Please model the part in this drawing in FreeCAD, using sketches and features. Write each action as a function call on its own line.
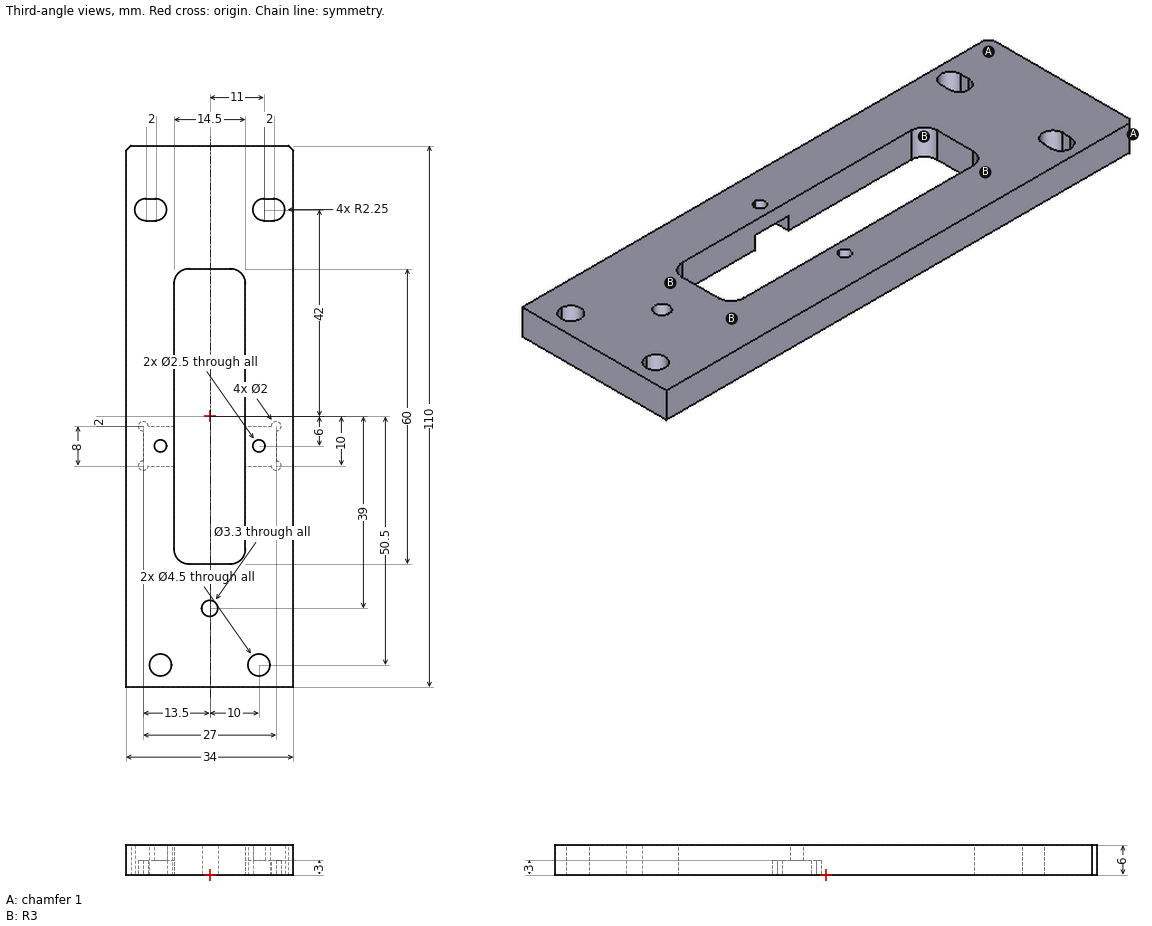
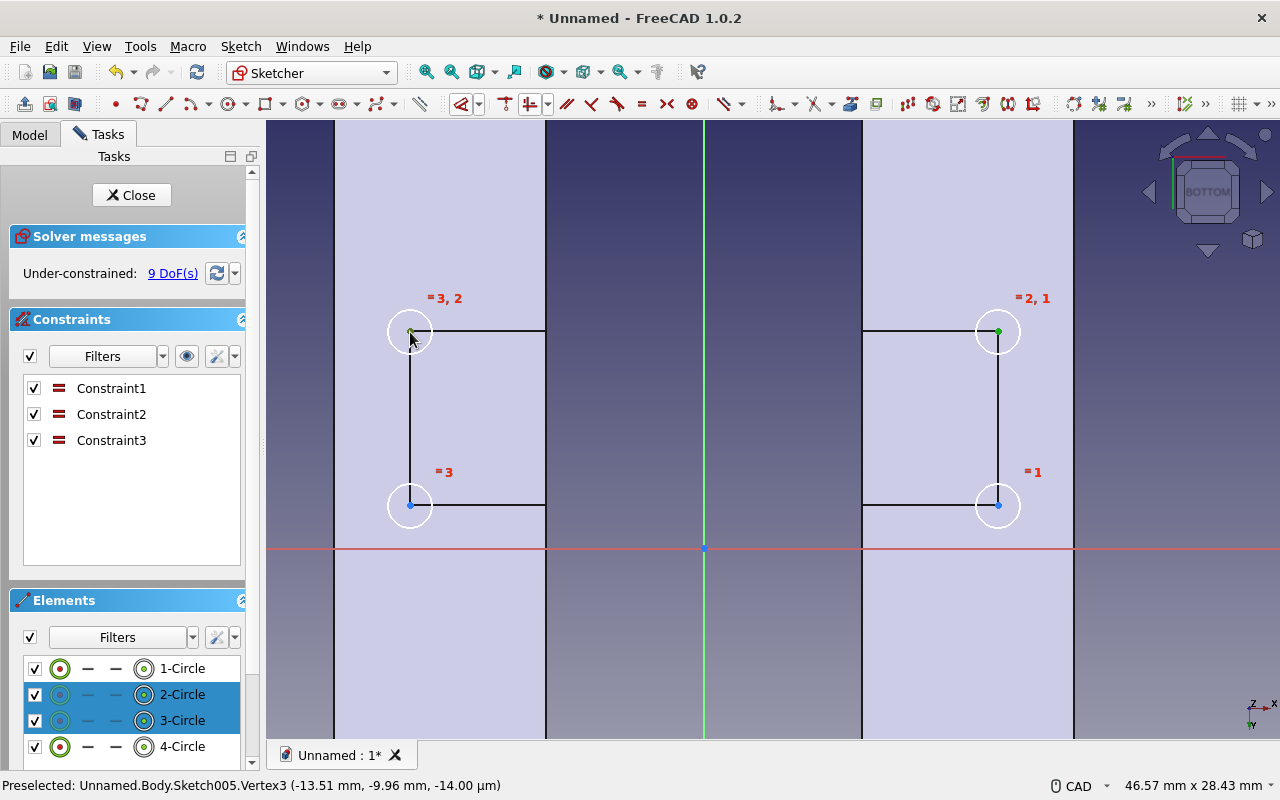
click(704, 671)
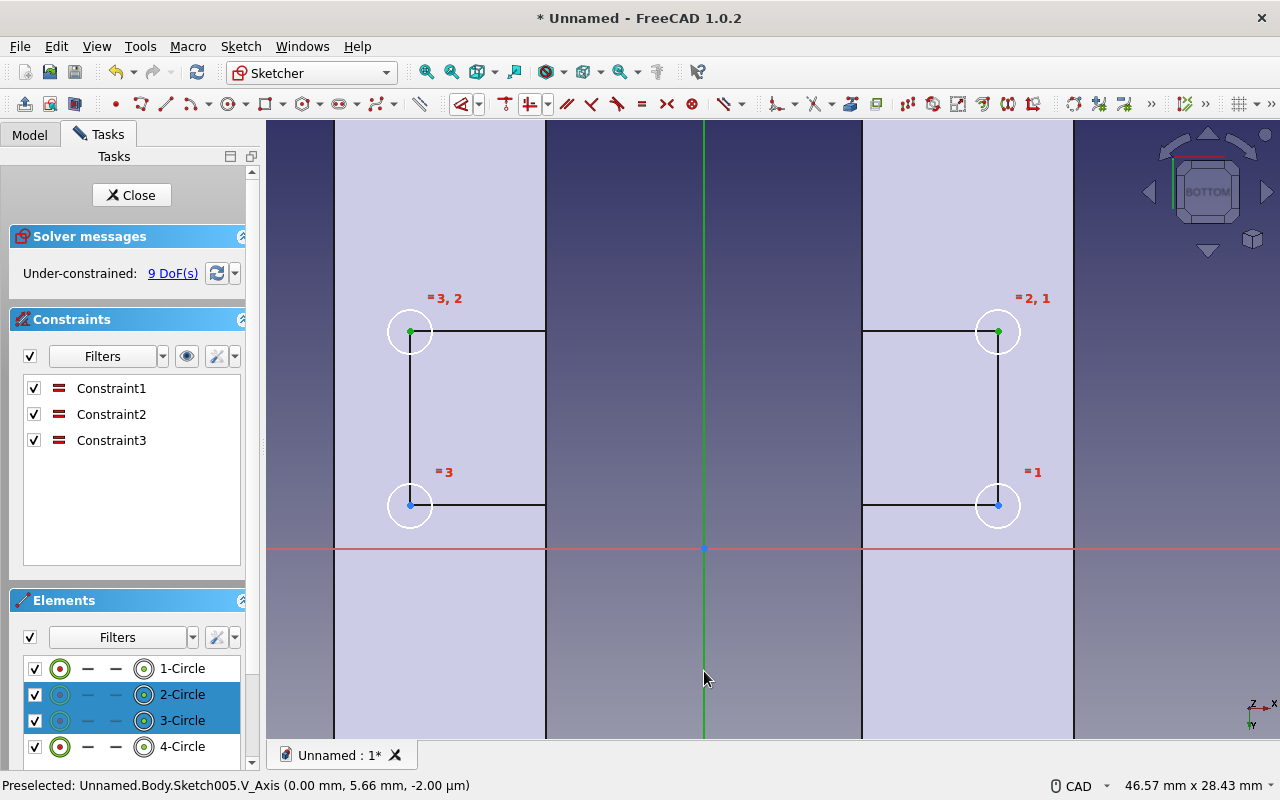
key(s)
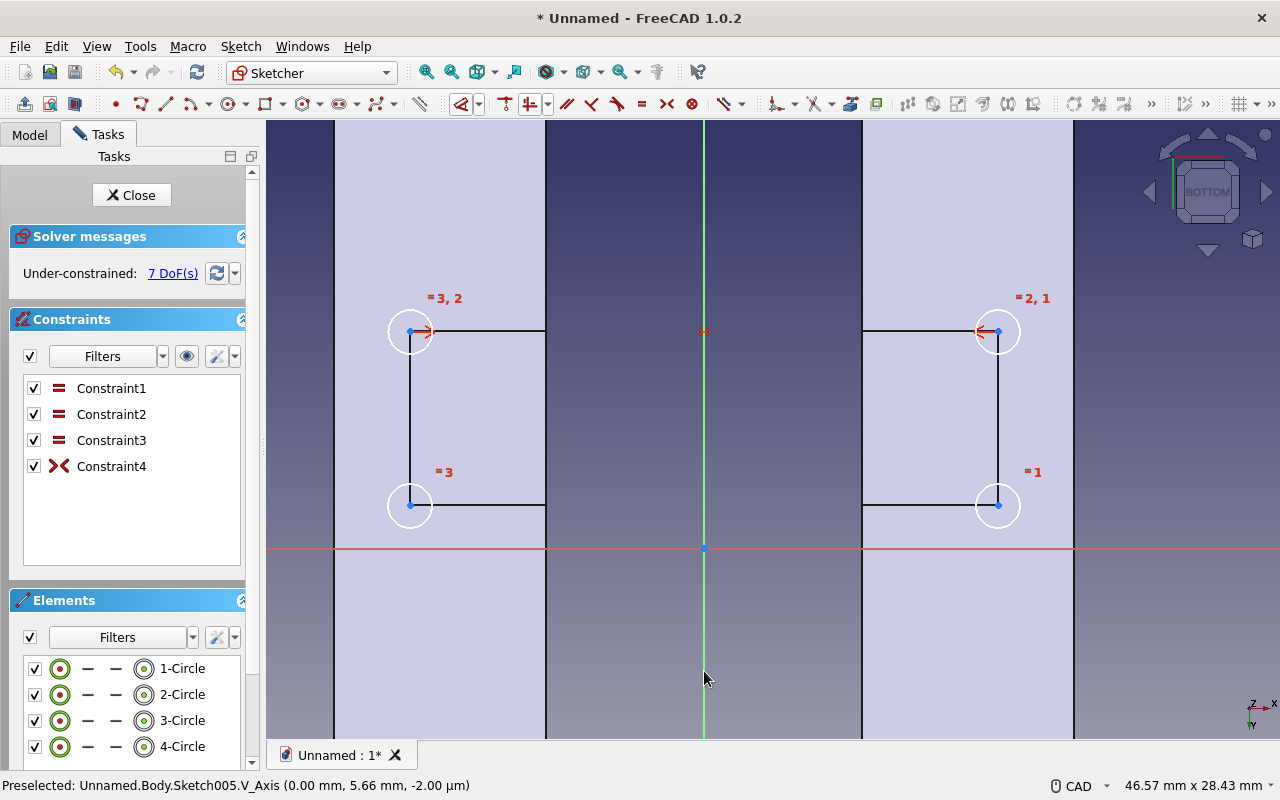
click(998, 506)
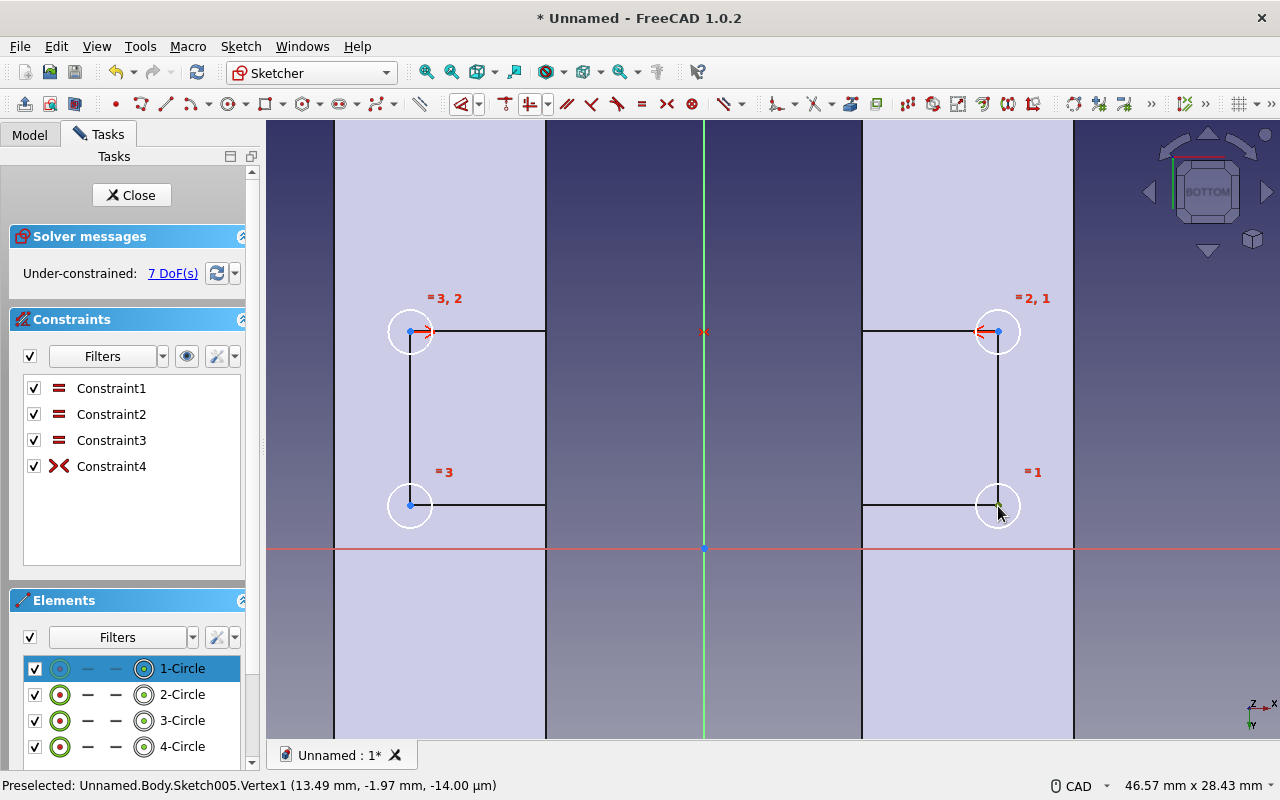
click(410, 506)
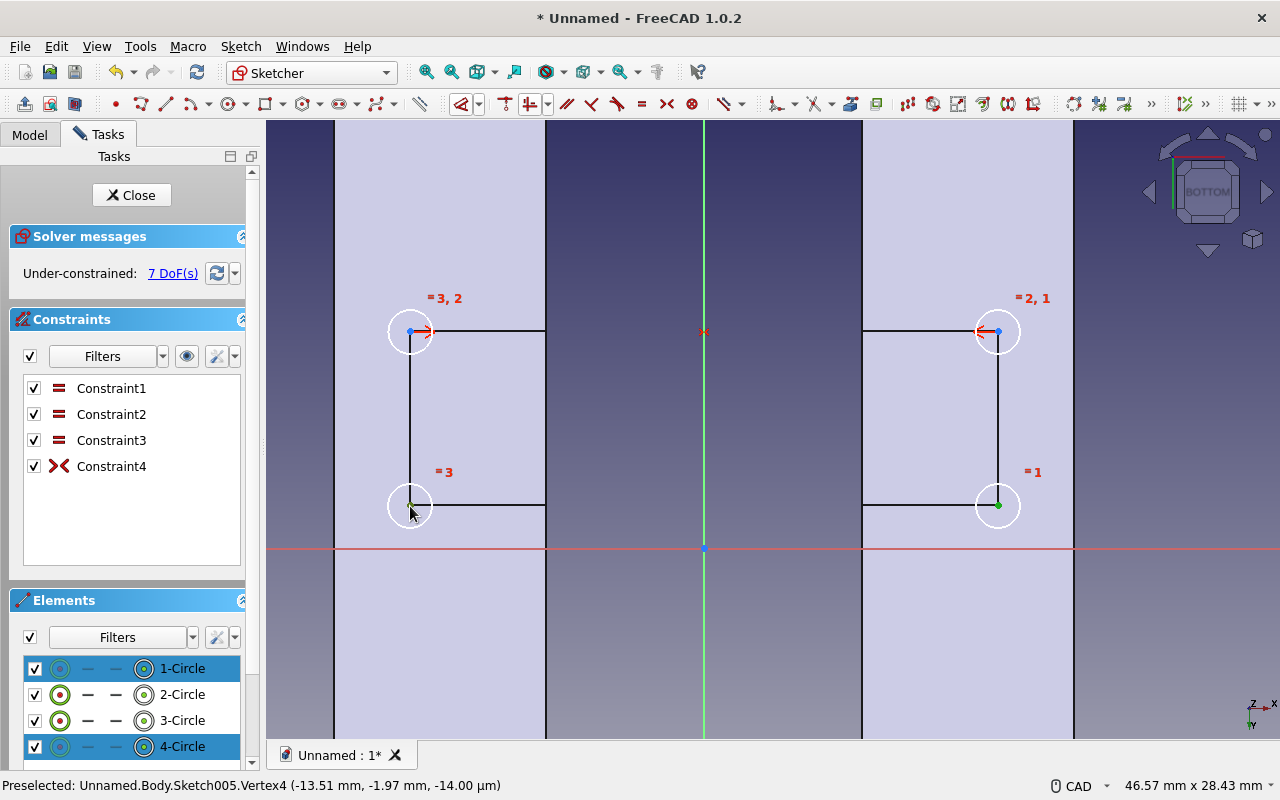
click(704, 671)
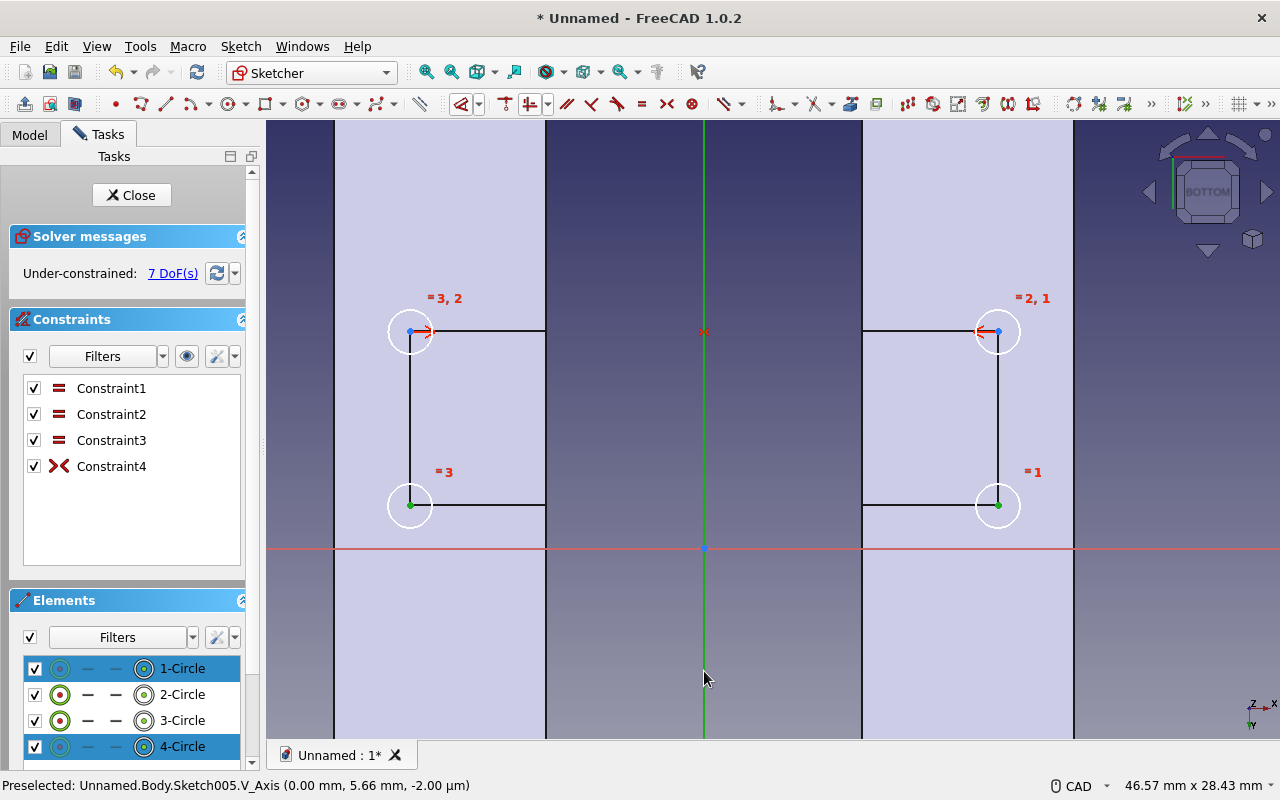
key(s)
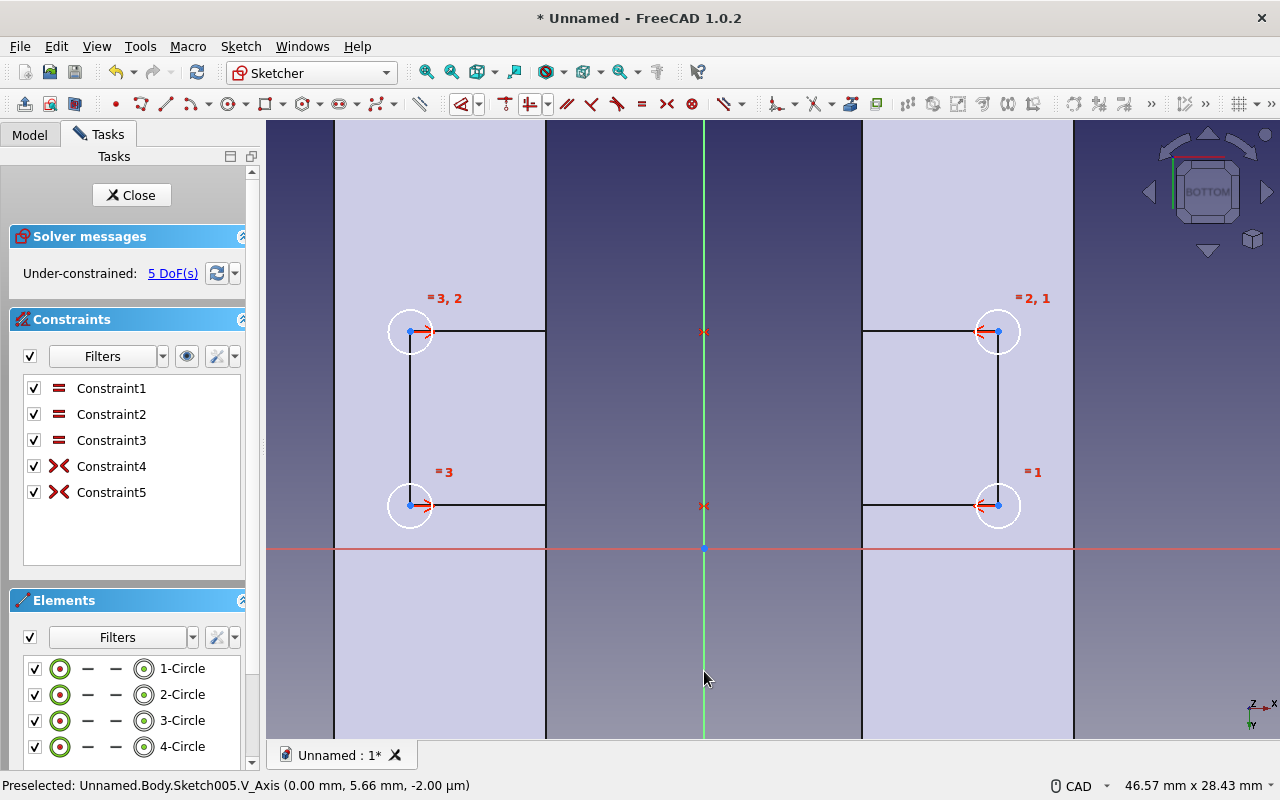
click(1014, 490)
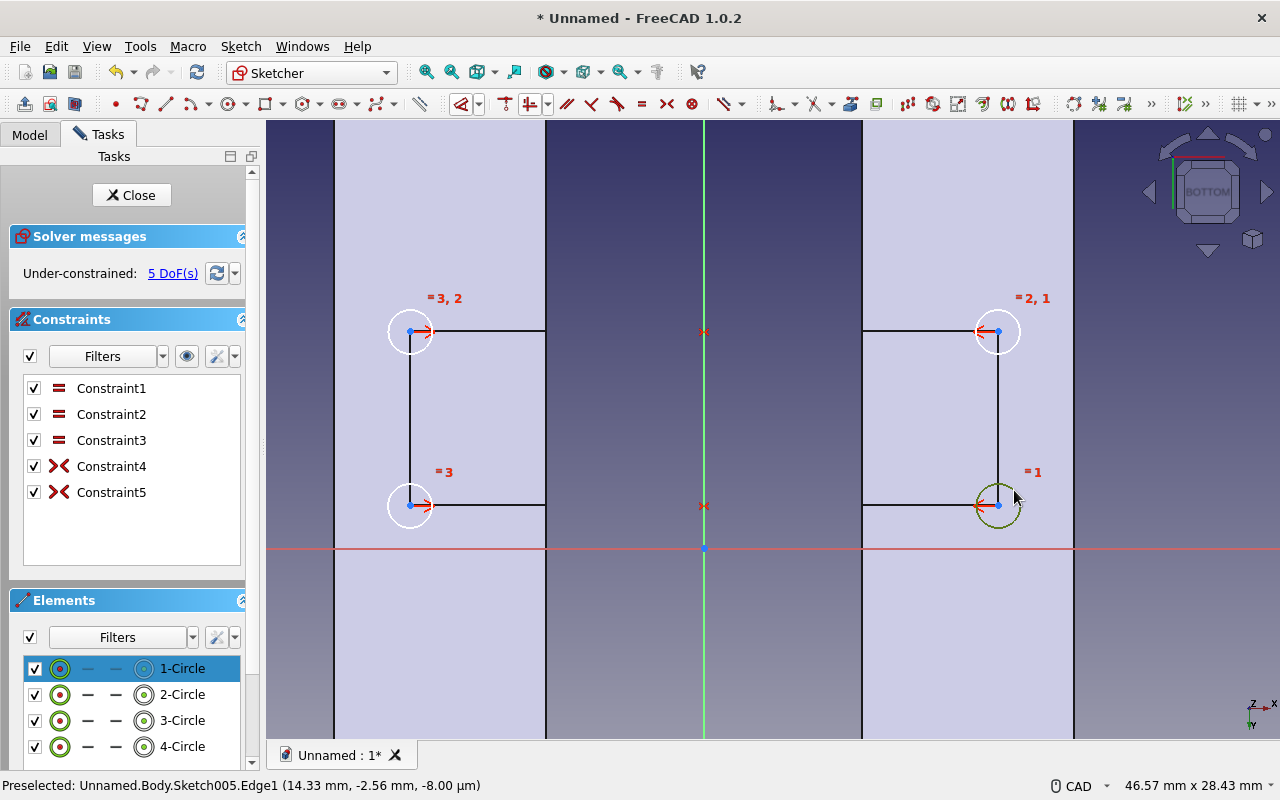
key(k)
key(o)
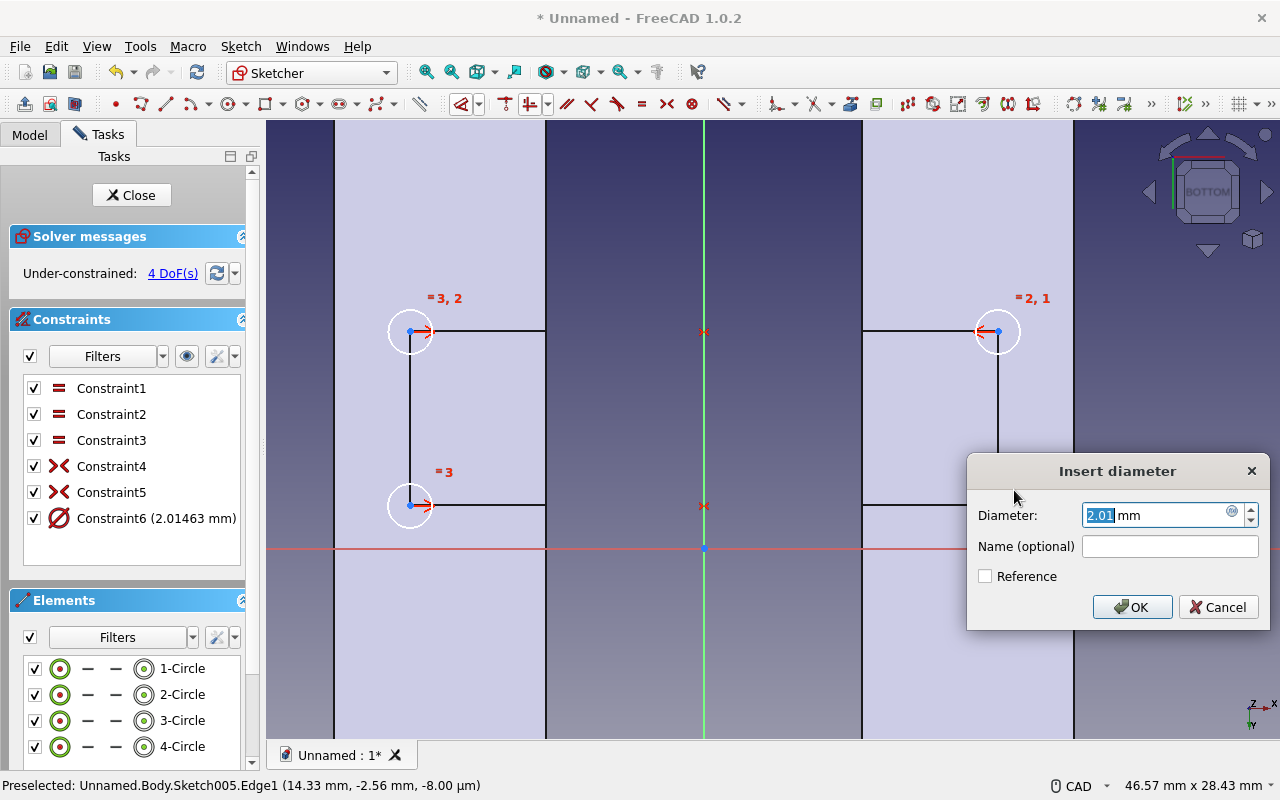
text(2)
key(Return)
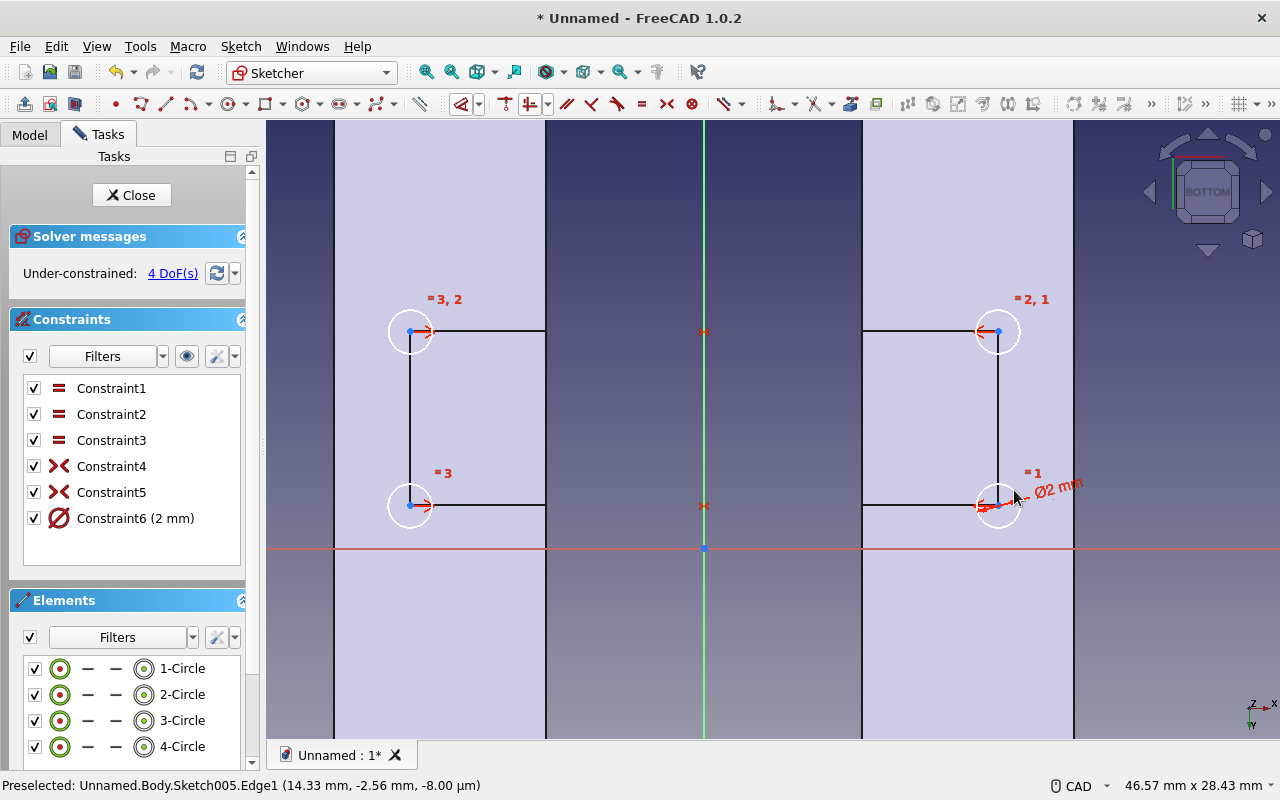
click(998, 506)